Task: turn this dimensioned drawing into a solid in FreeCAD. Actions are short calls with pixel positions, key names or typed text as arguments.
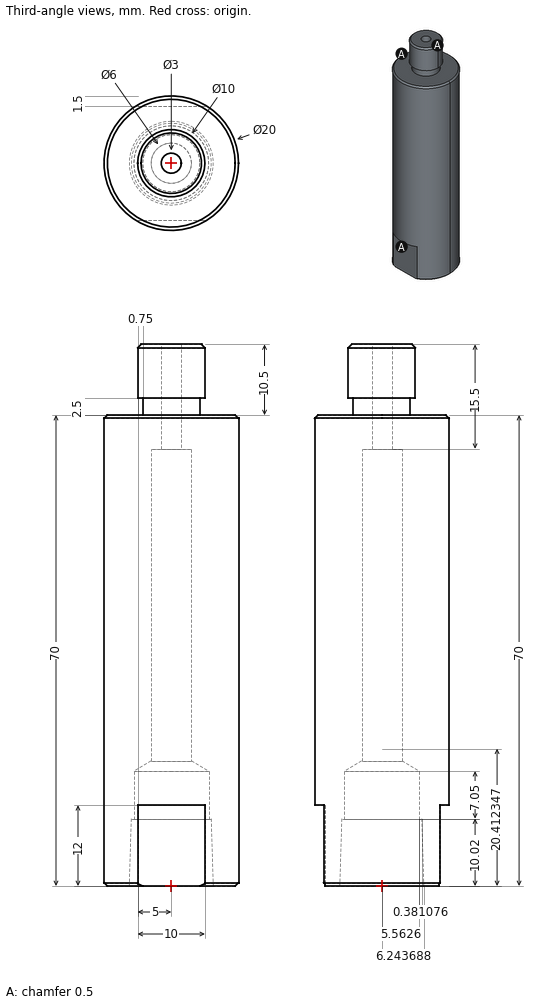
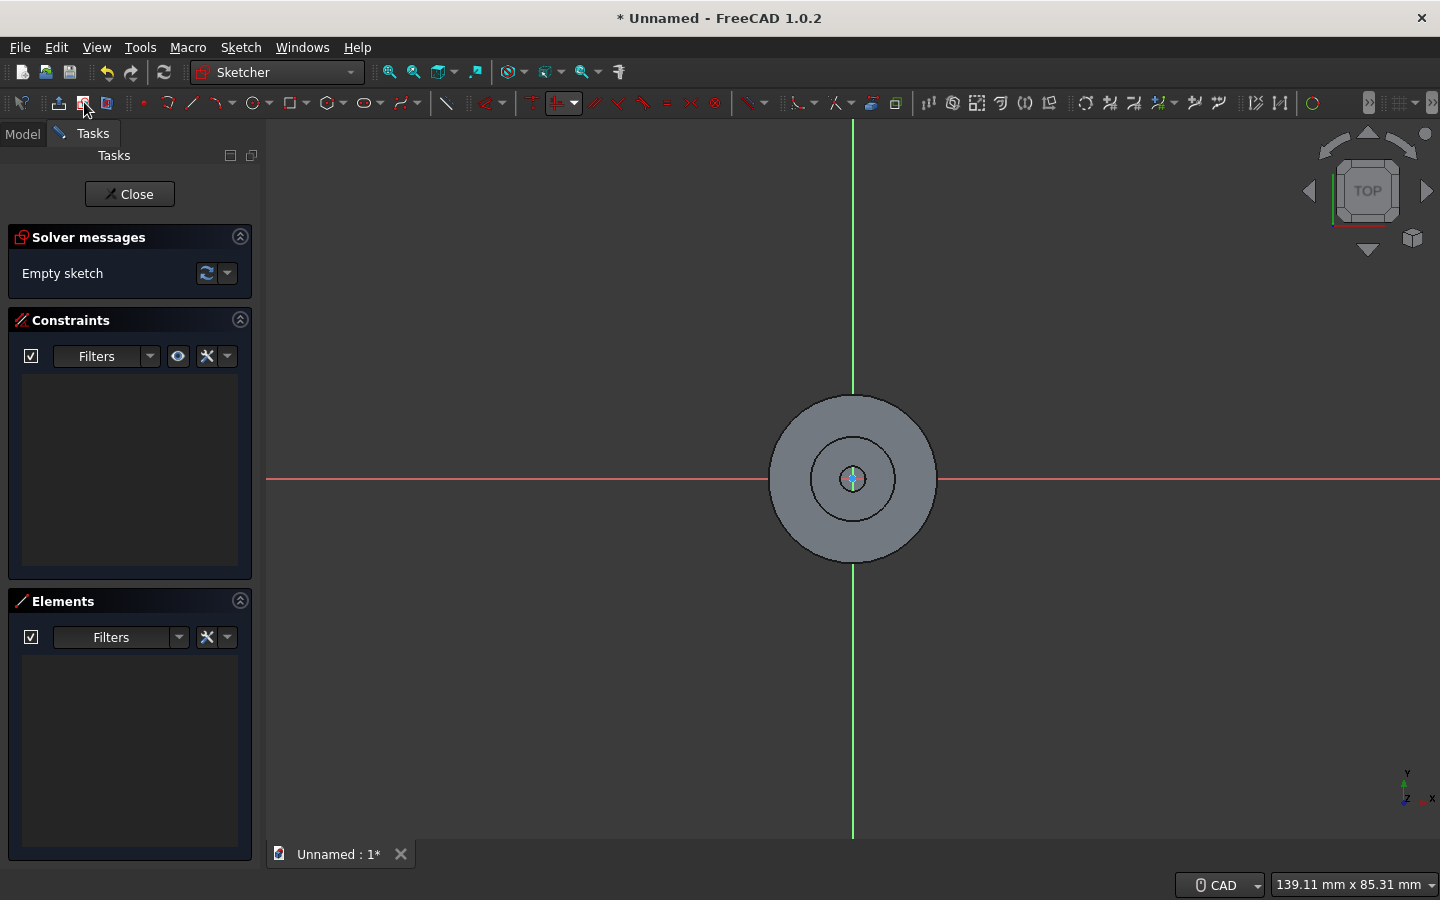
click(108, 104)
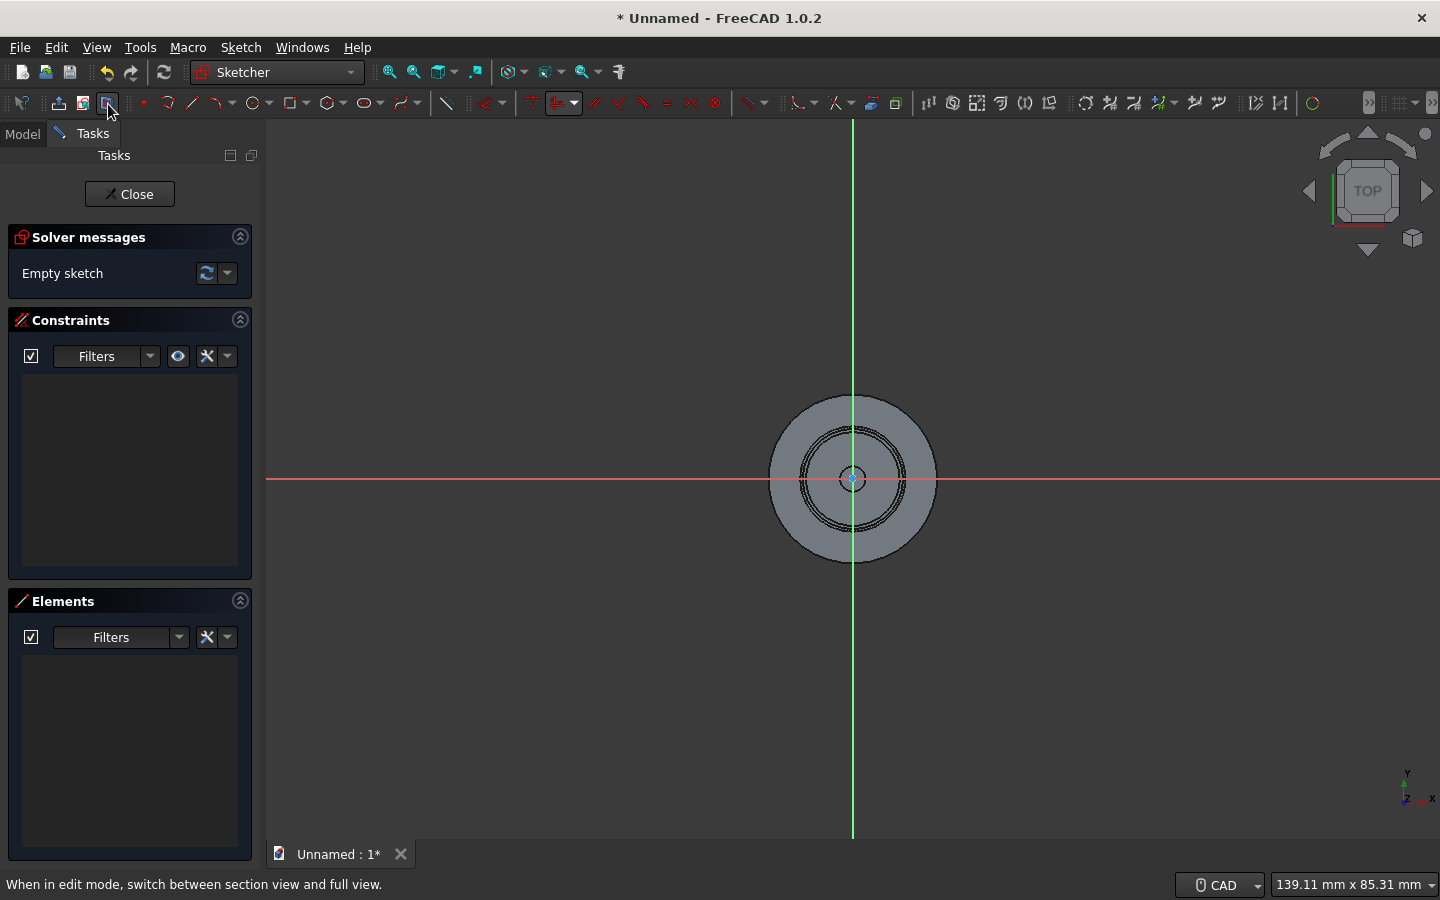
scroll(861, 479, up, 11)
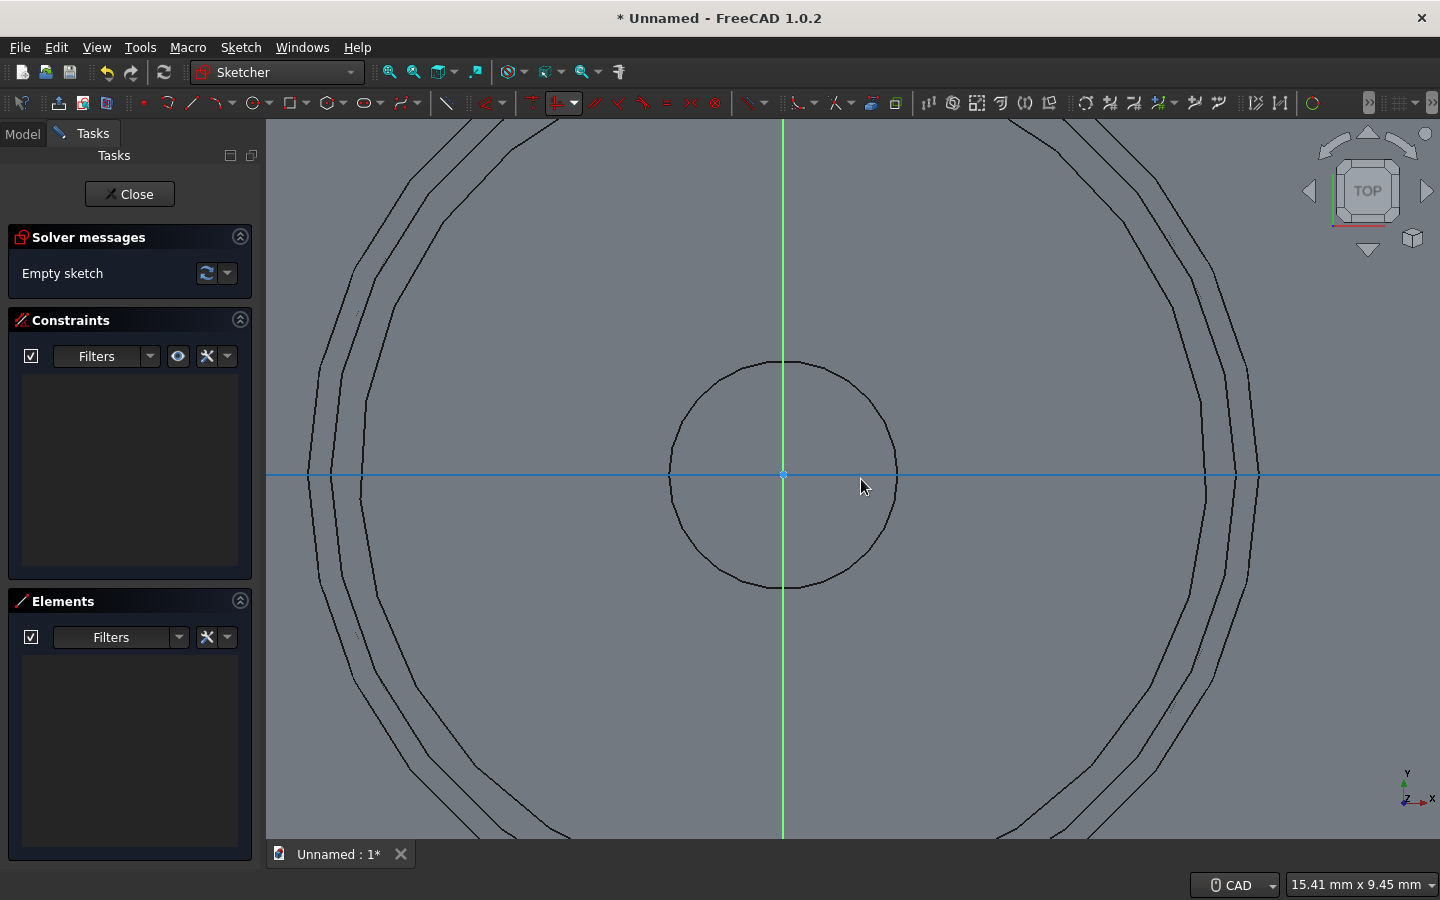
key(g)
key(c)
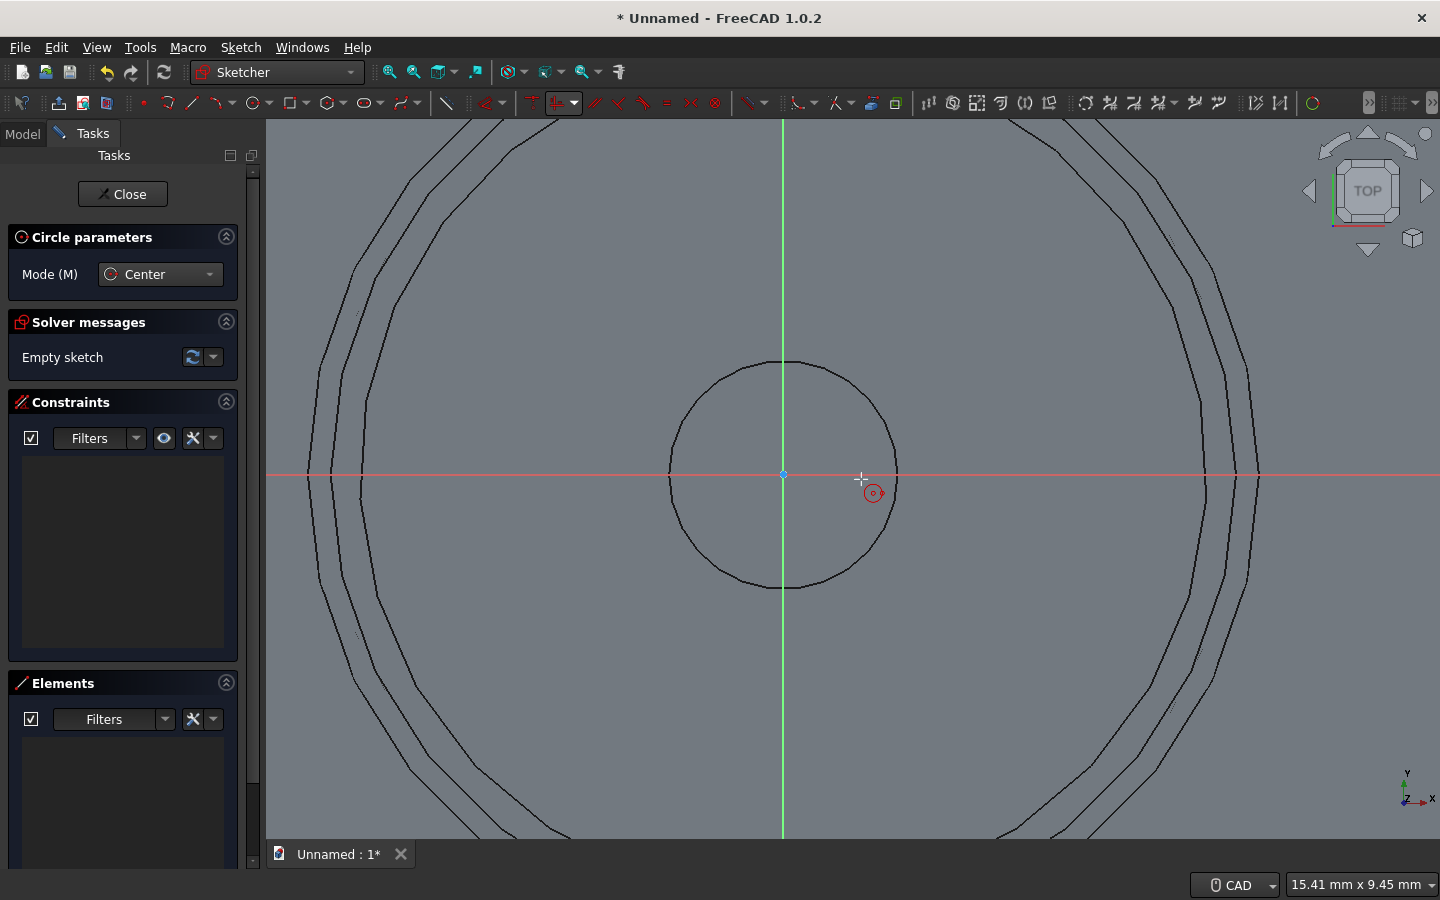
click(783, 475)
move(945, 313)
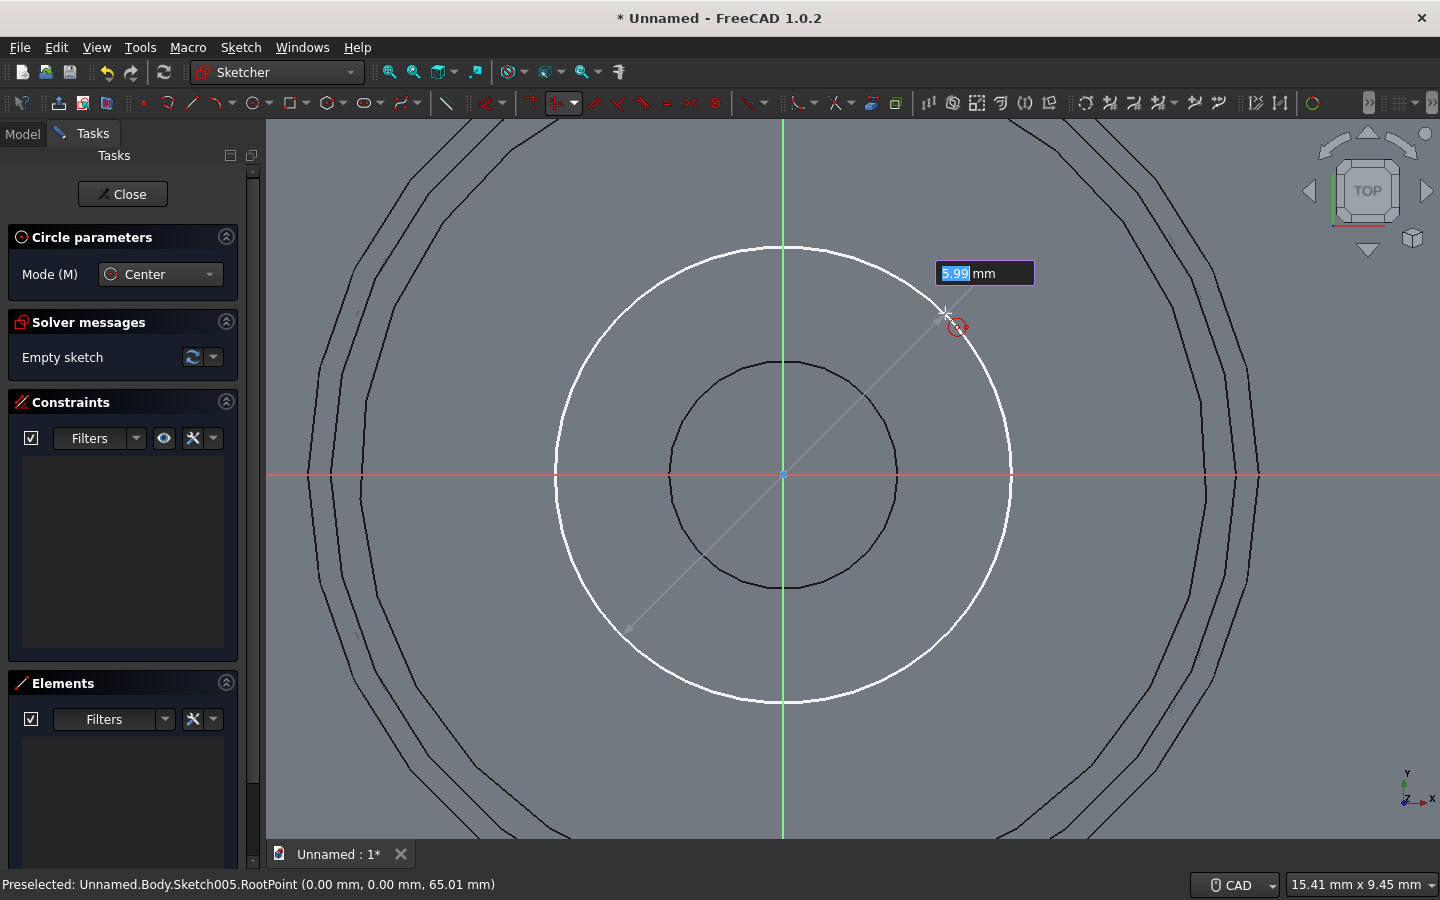
text(6)
key(Return)
key(Escape)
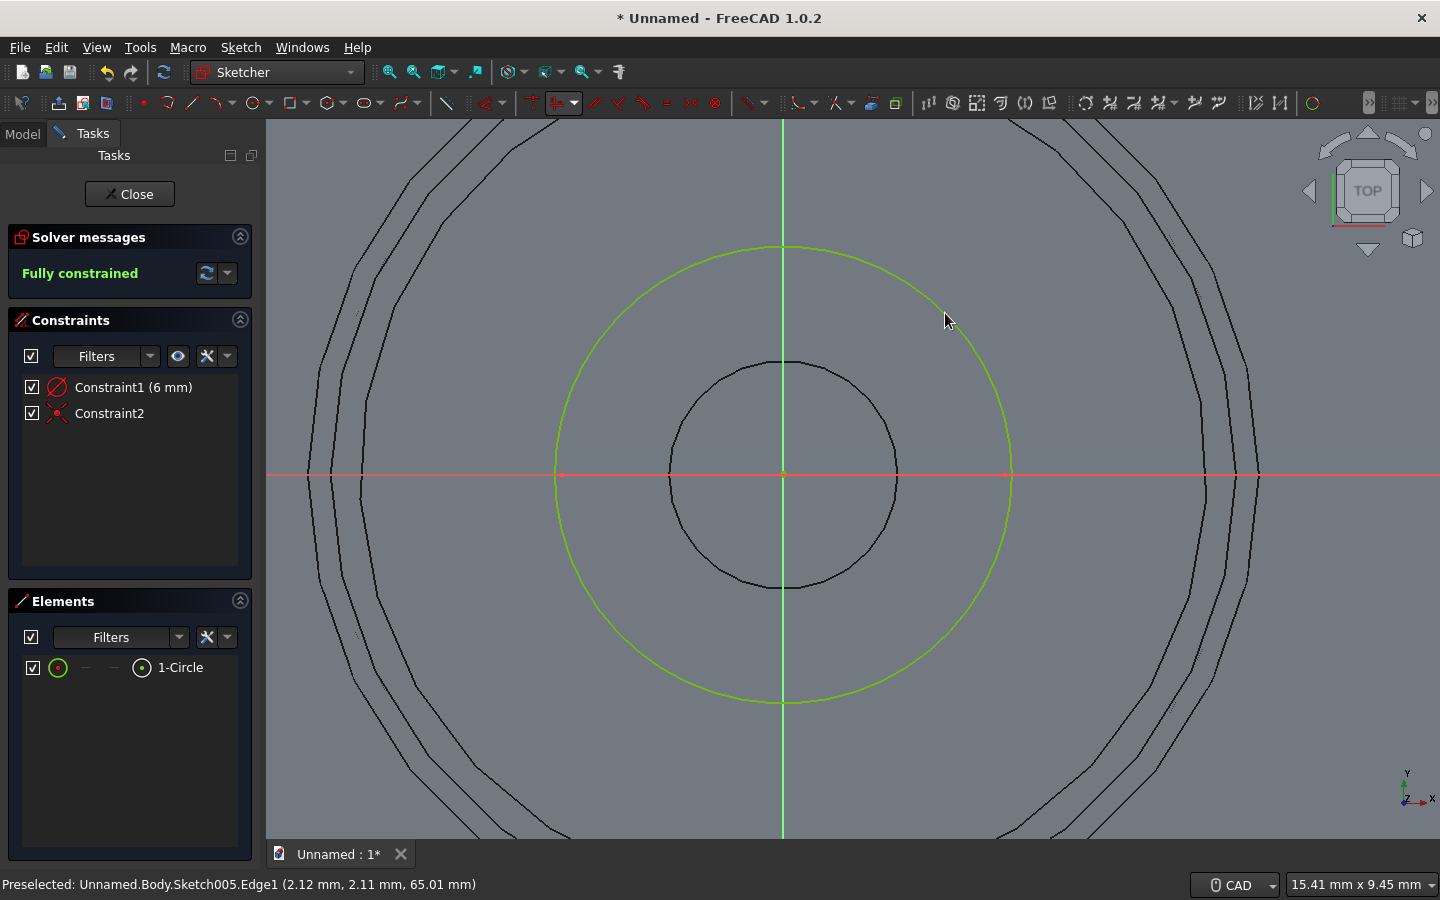
click(130, 194)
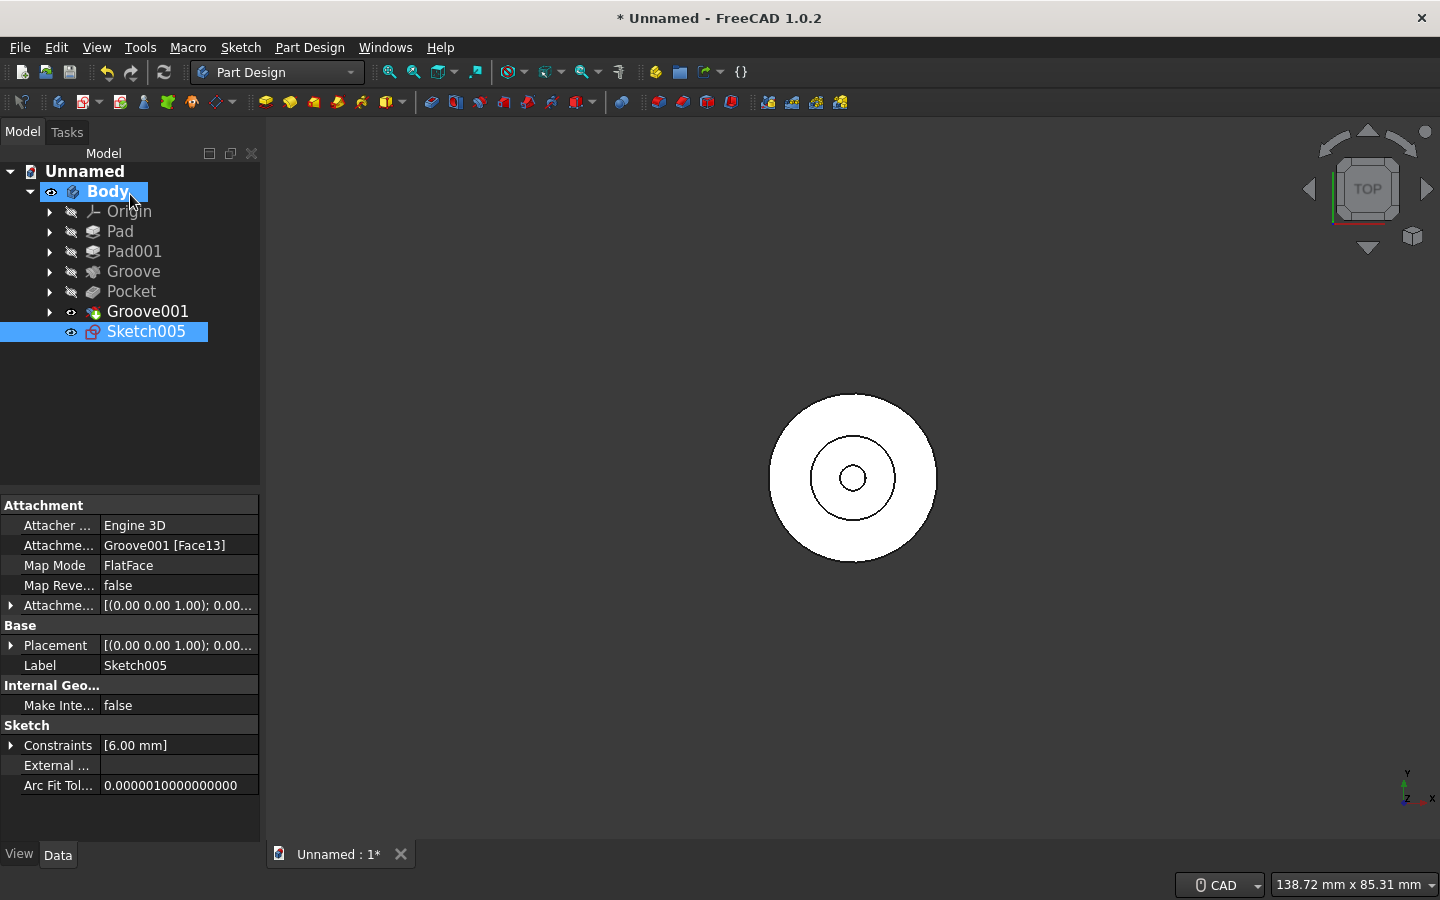
click(432, 102)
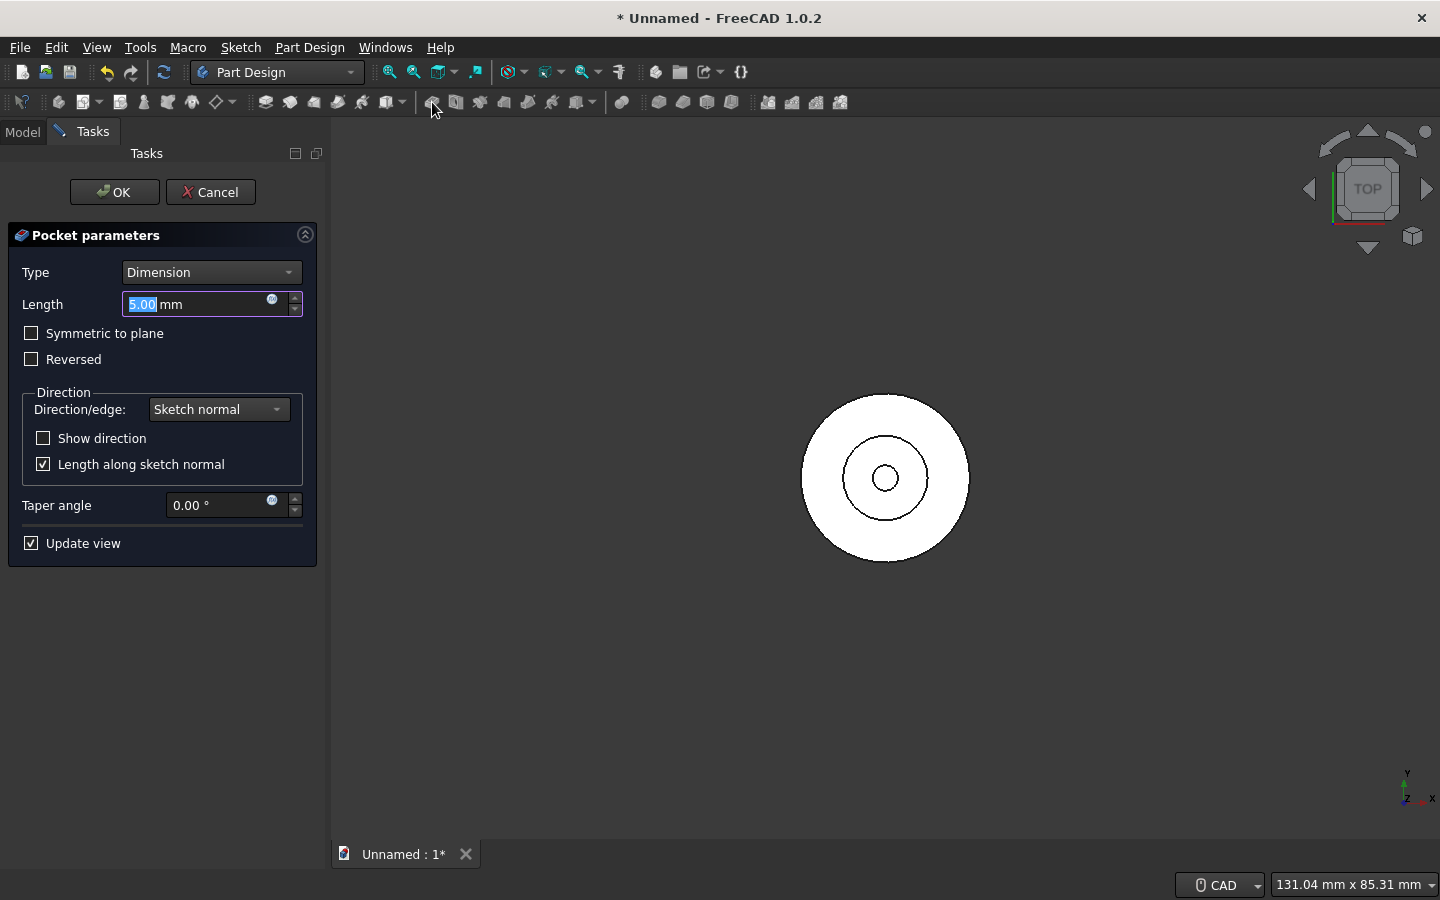
click(212, 272)